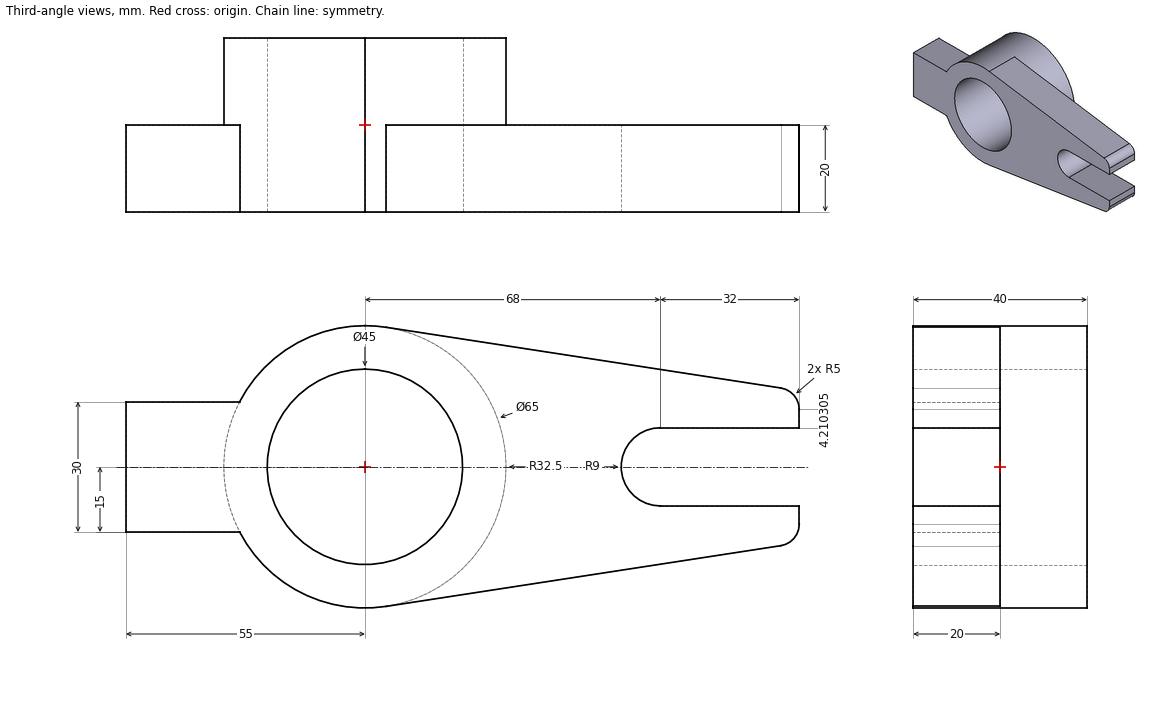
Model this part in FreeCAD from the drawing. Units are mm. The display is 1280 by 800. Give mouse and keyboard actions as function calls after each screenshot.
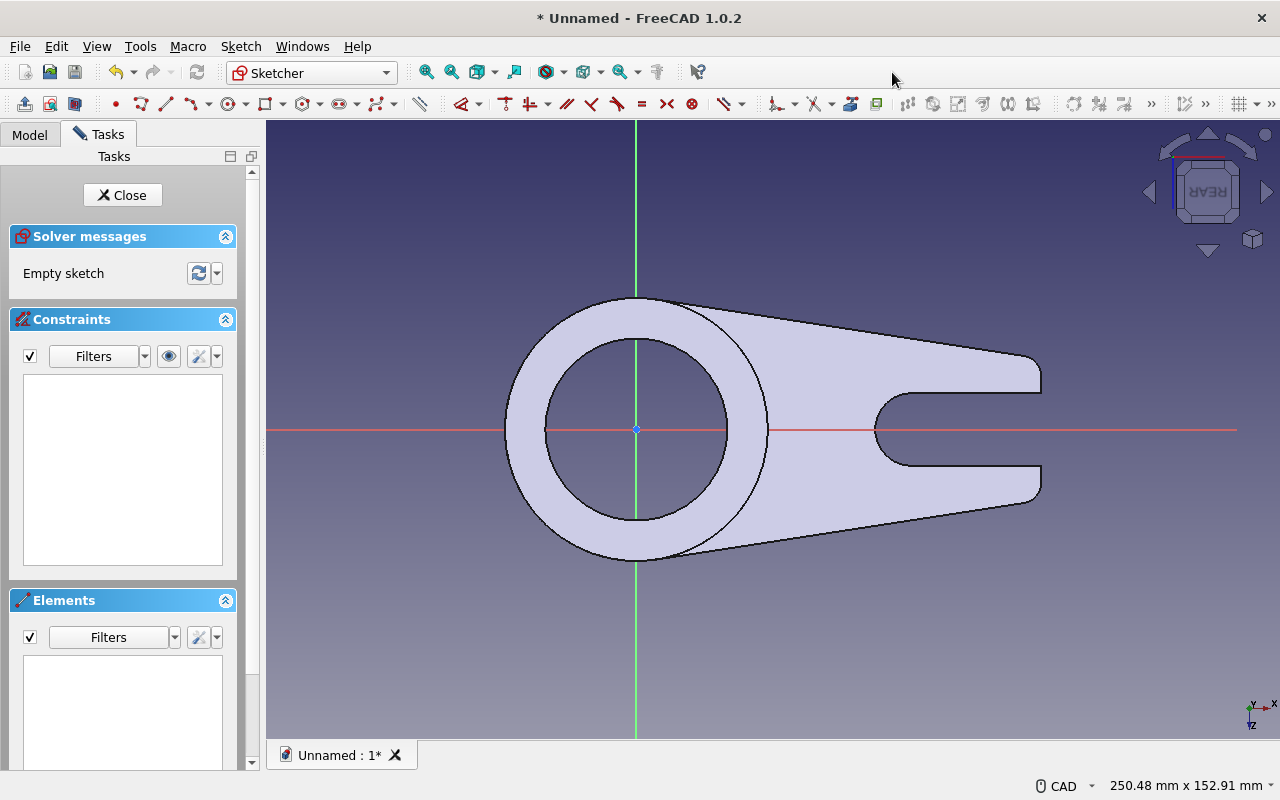
key(q)
key(s)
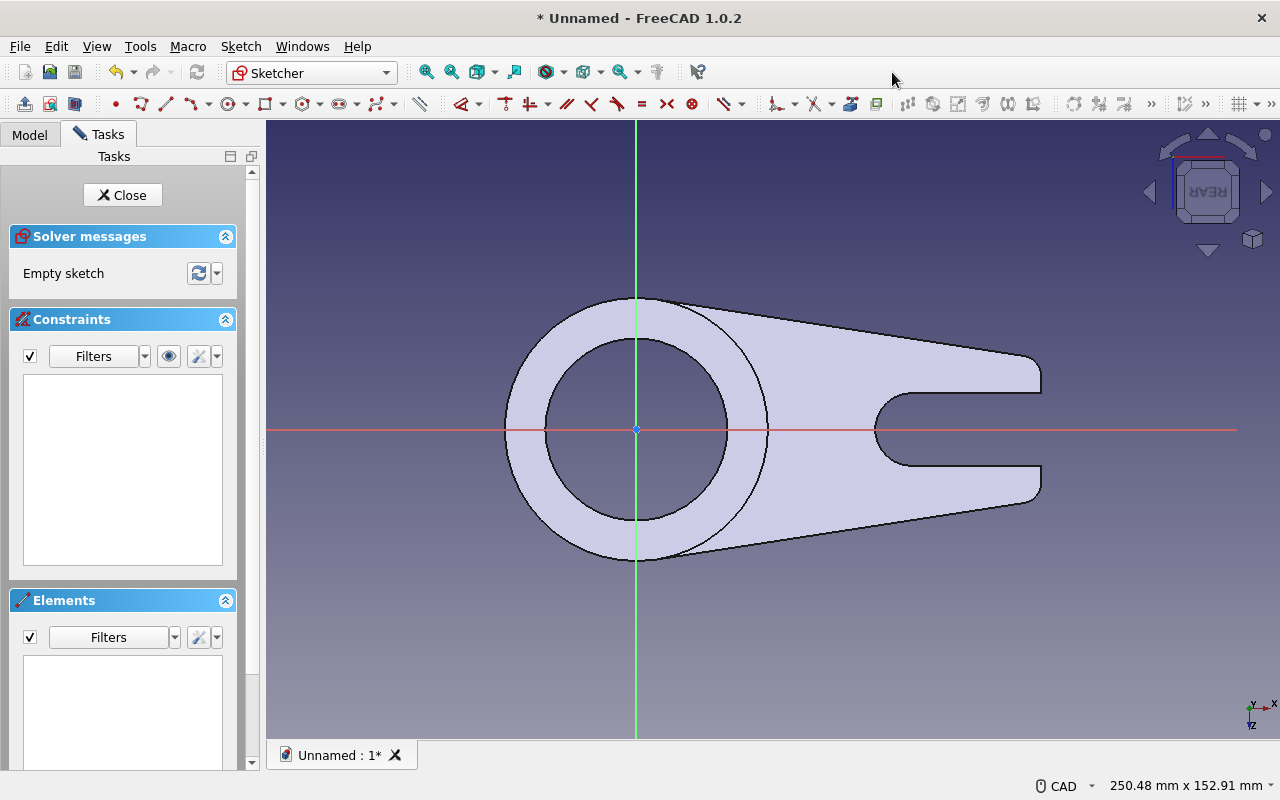
scroll(421, 429, up, 5)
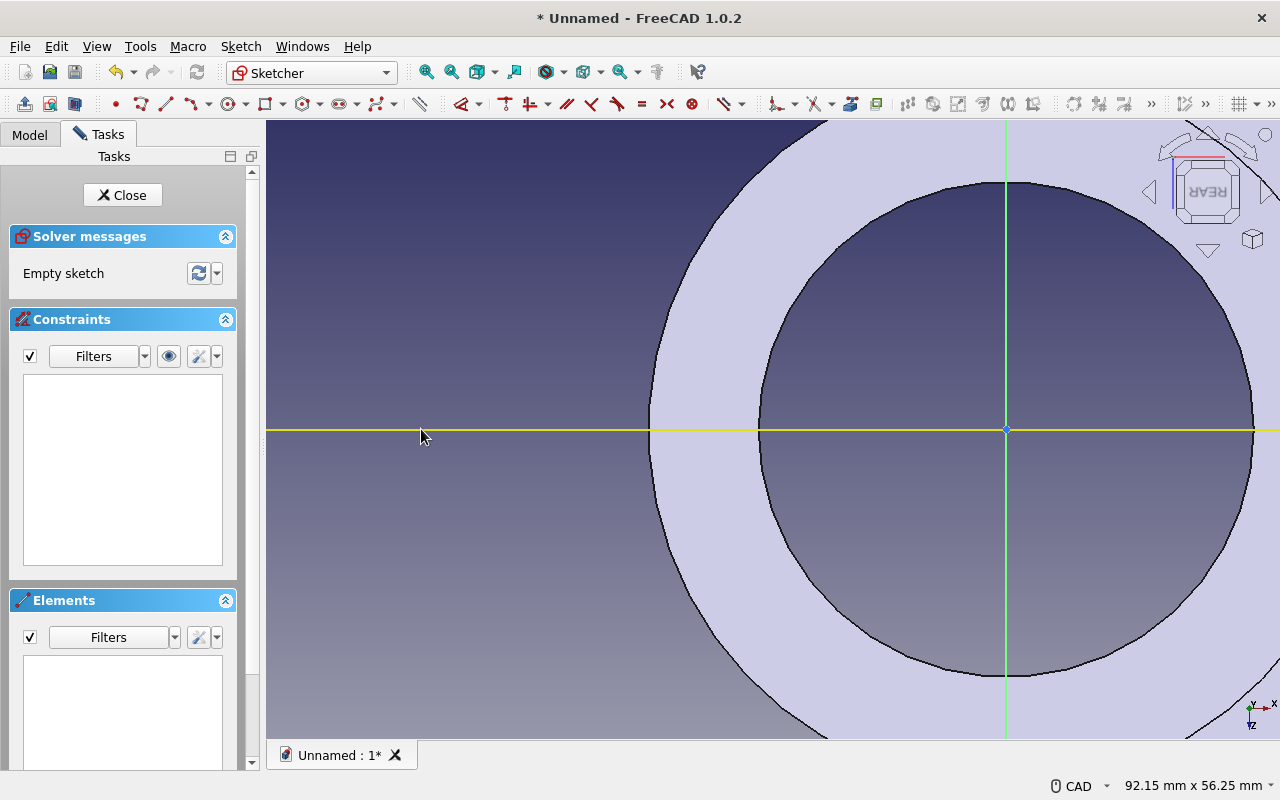
key(g)
key(m)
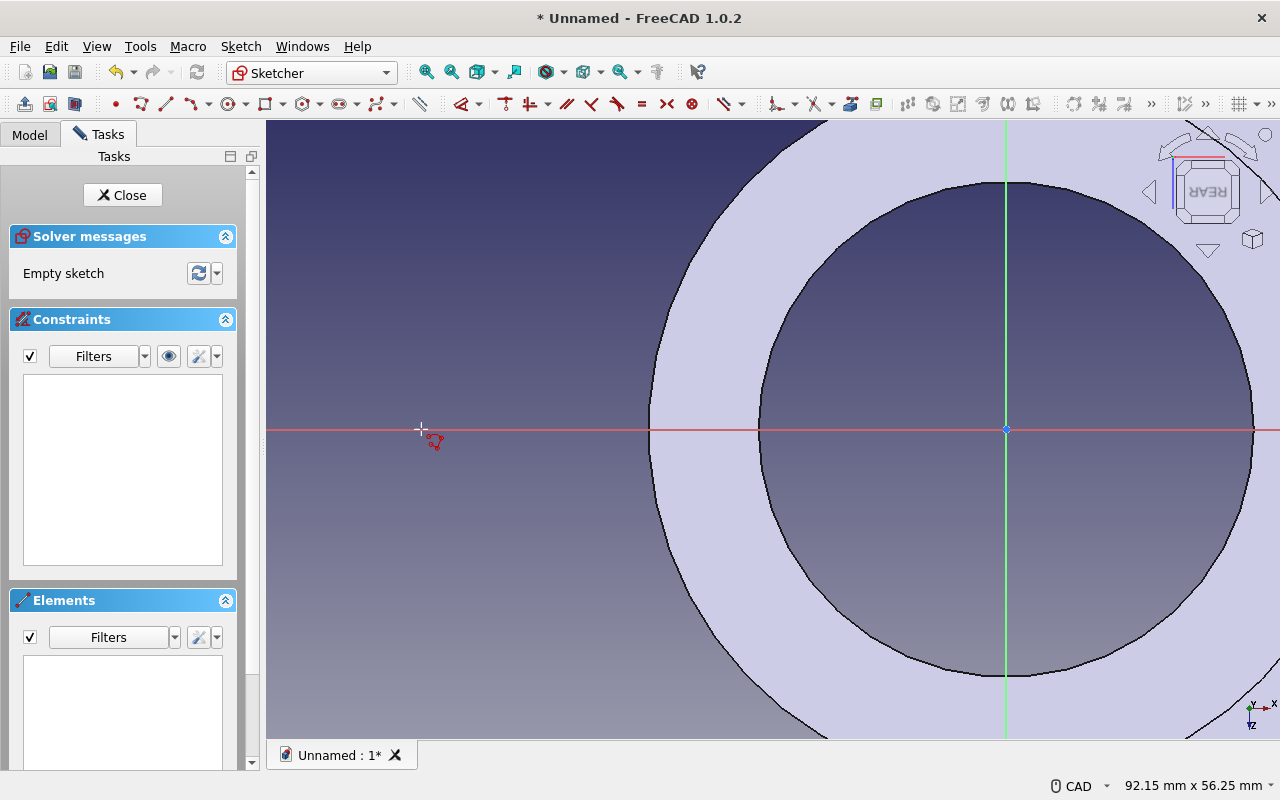
click(689, 264)
click(401, 264)
click(401, 595)
click(689, 595)
right_click(689, 595)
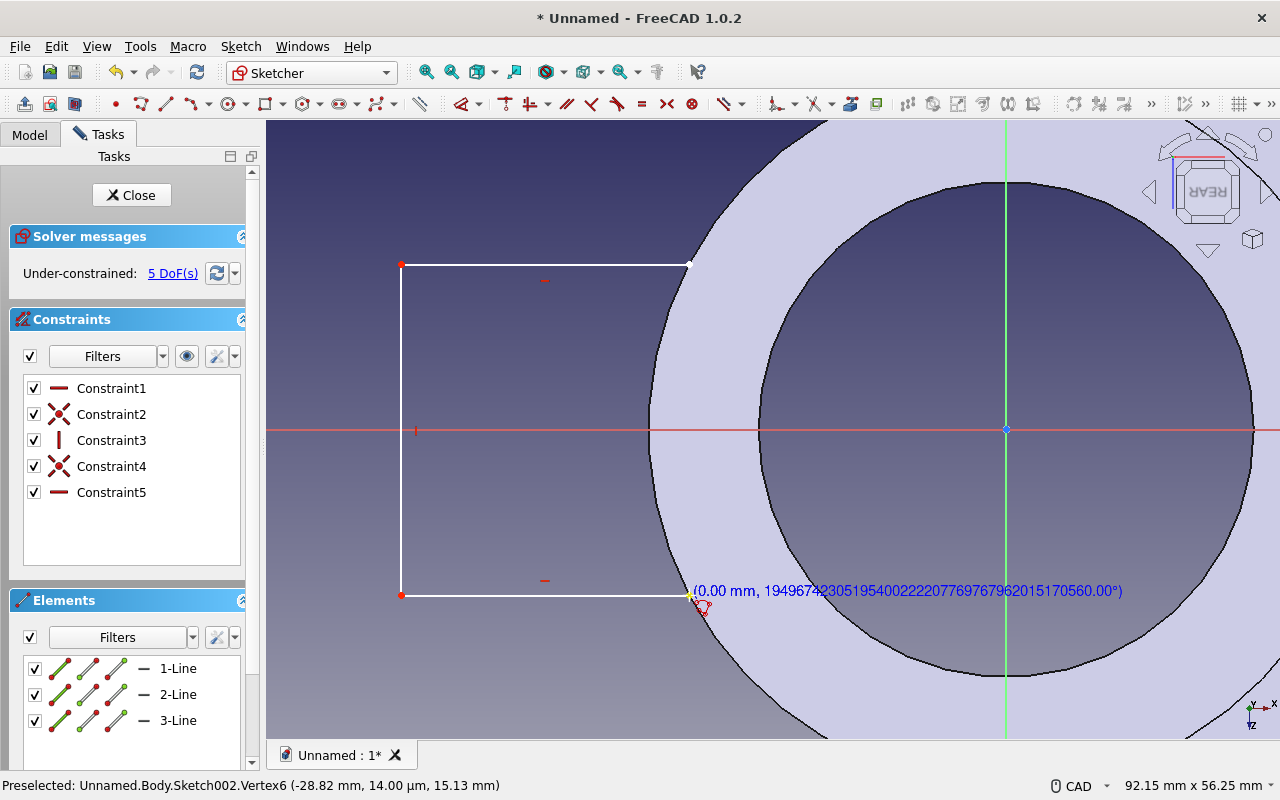
click(190, 104)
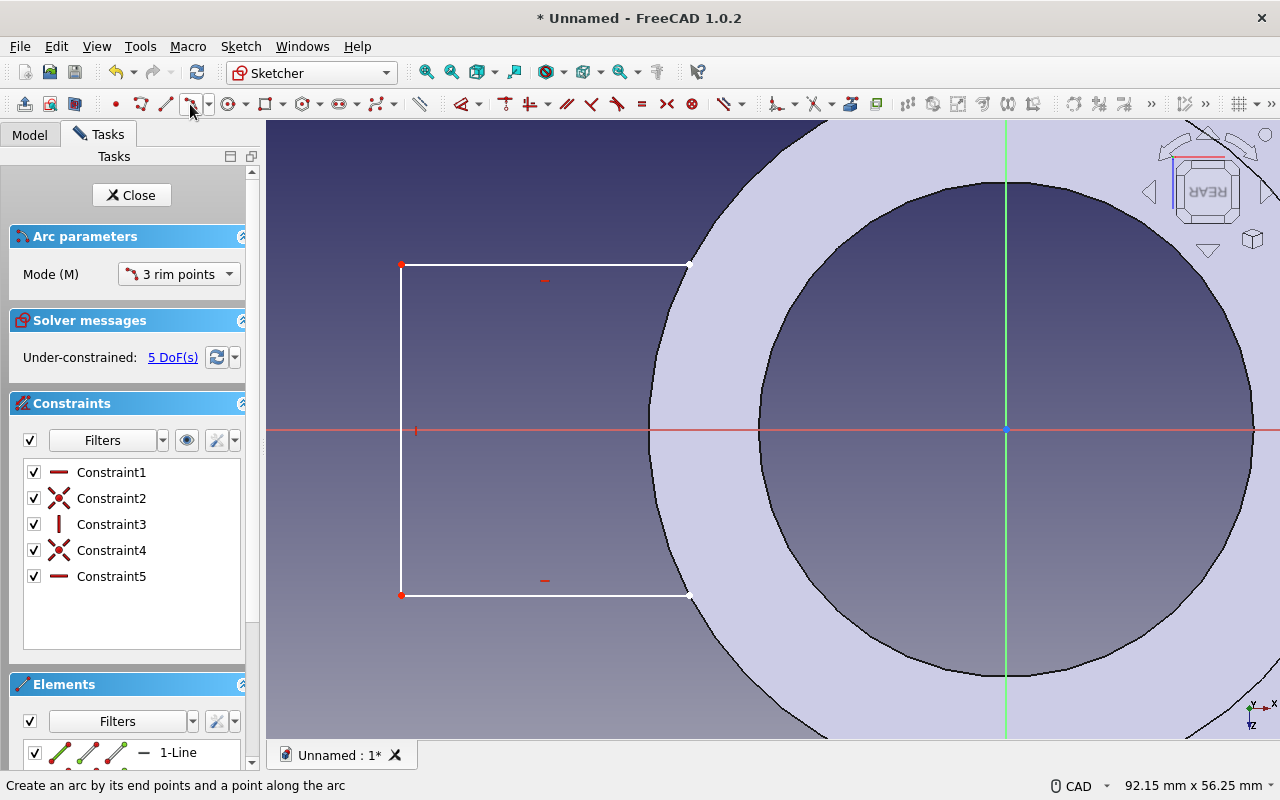
click(689, 596)
click(689, 265)
click(650, 395)
key(Escape)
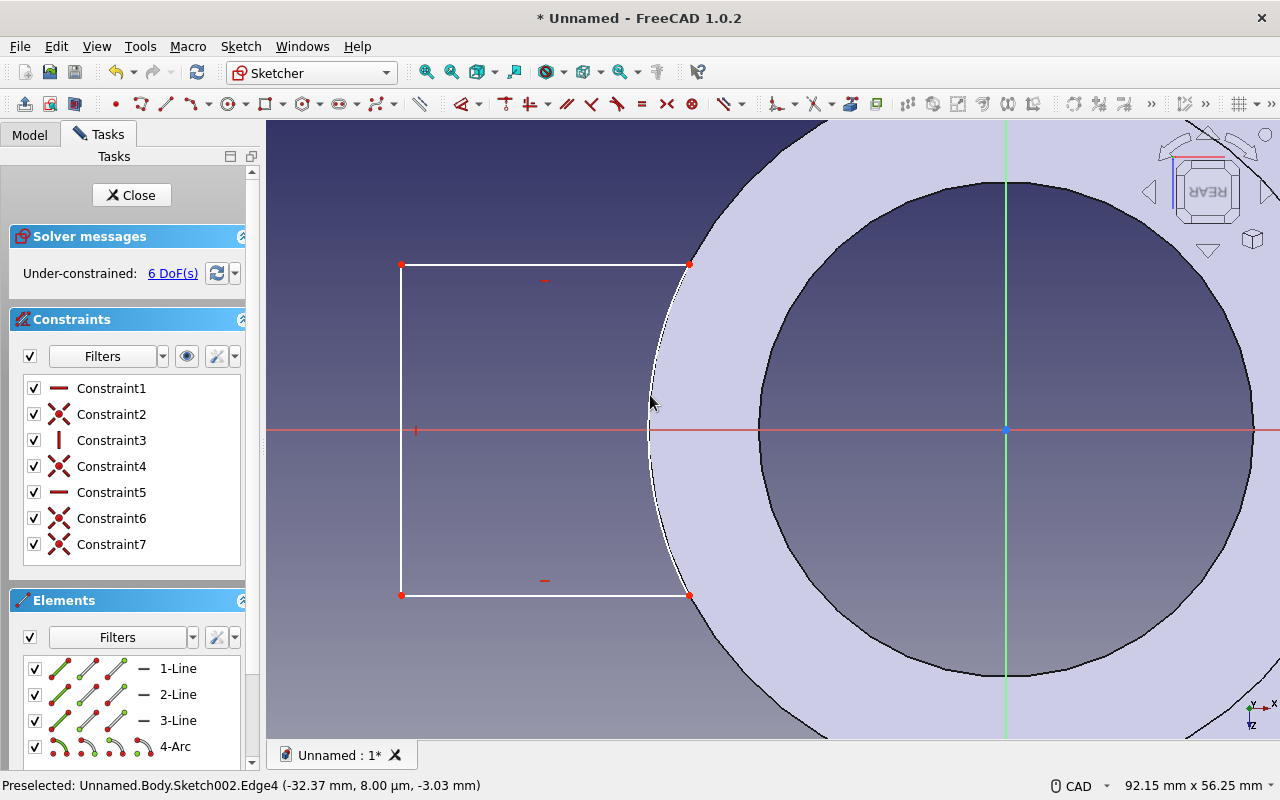
drag(995, 419, 1016, 441)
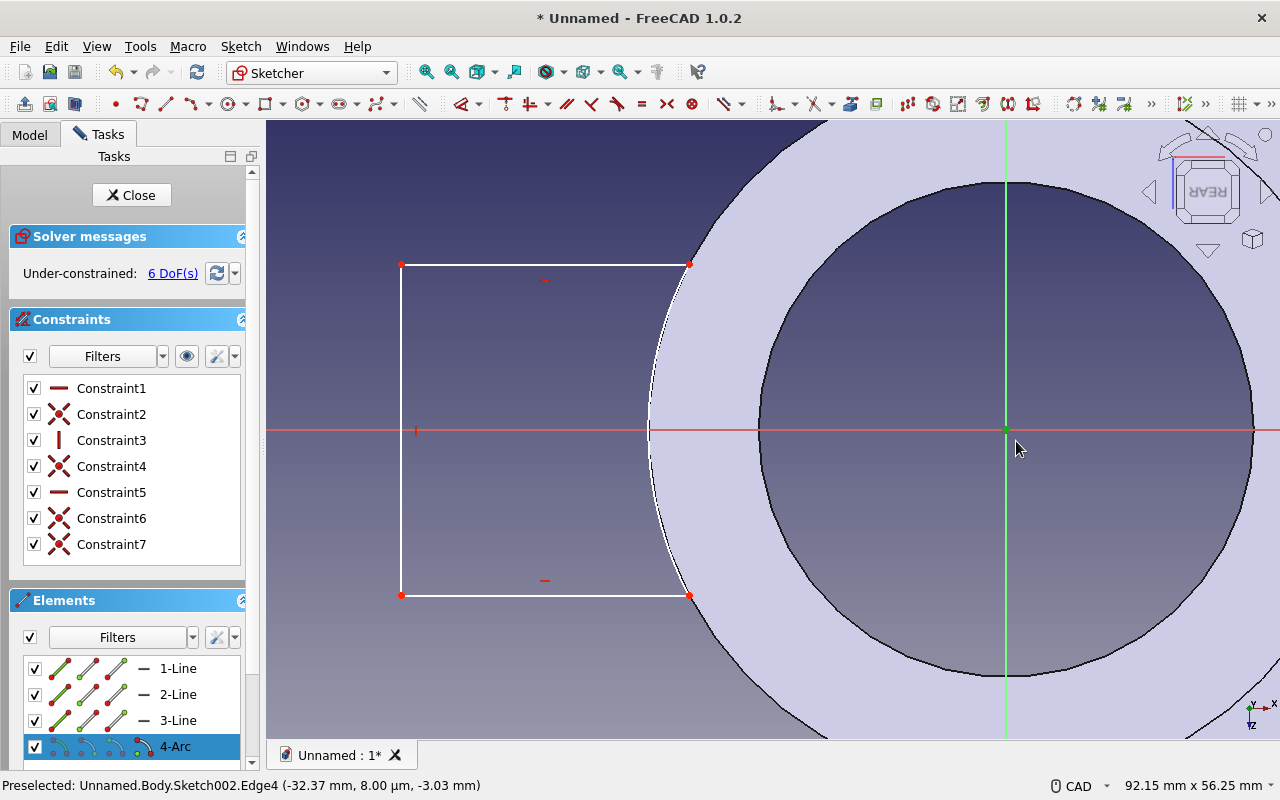
key(c)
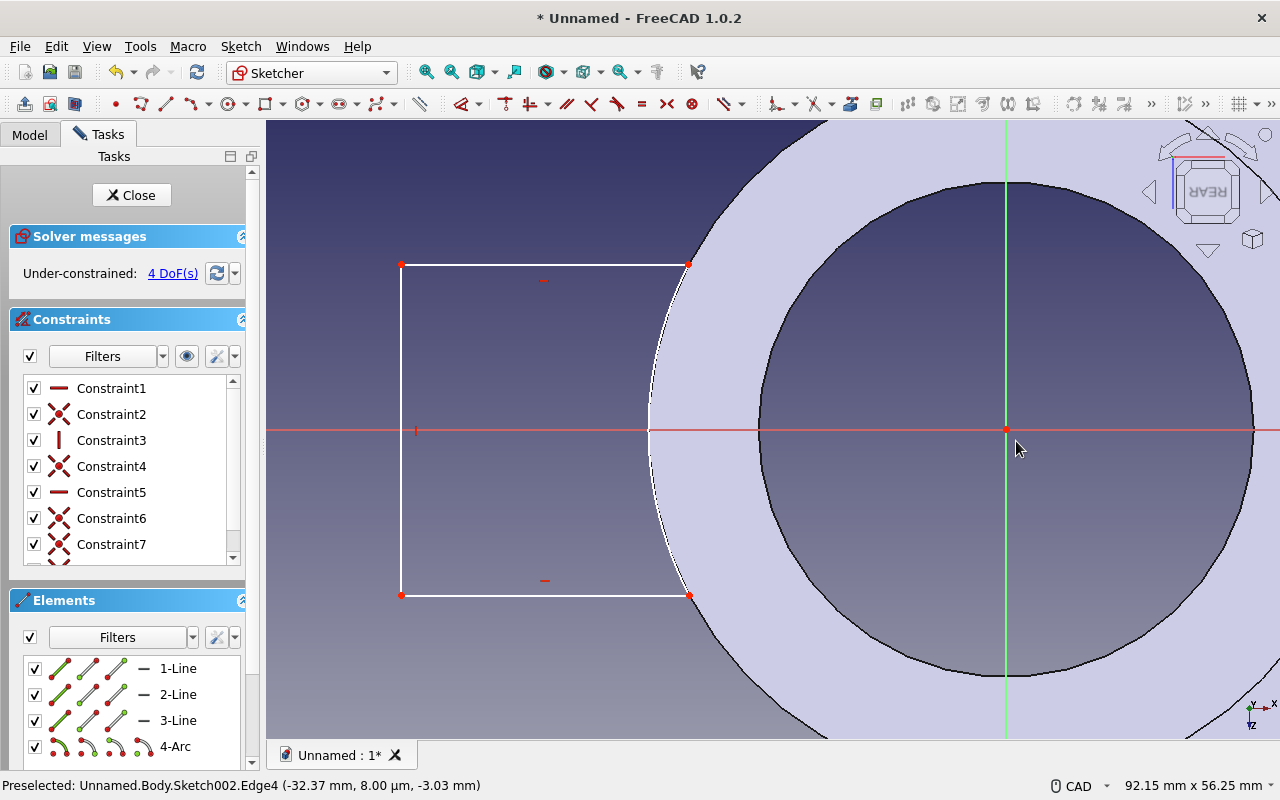
key(d)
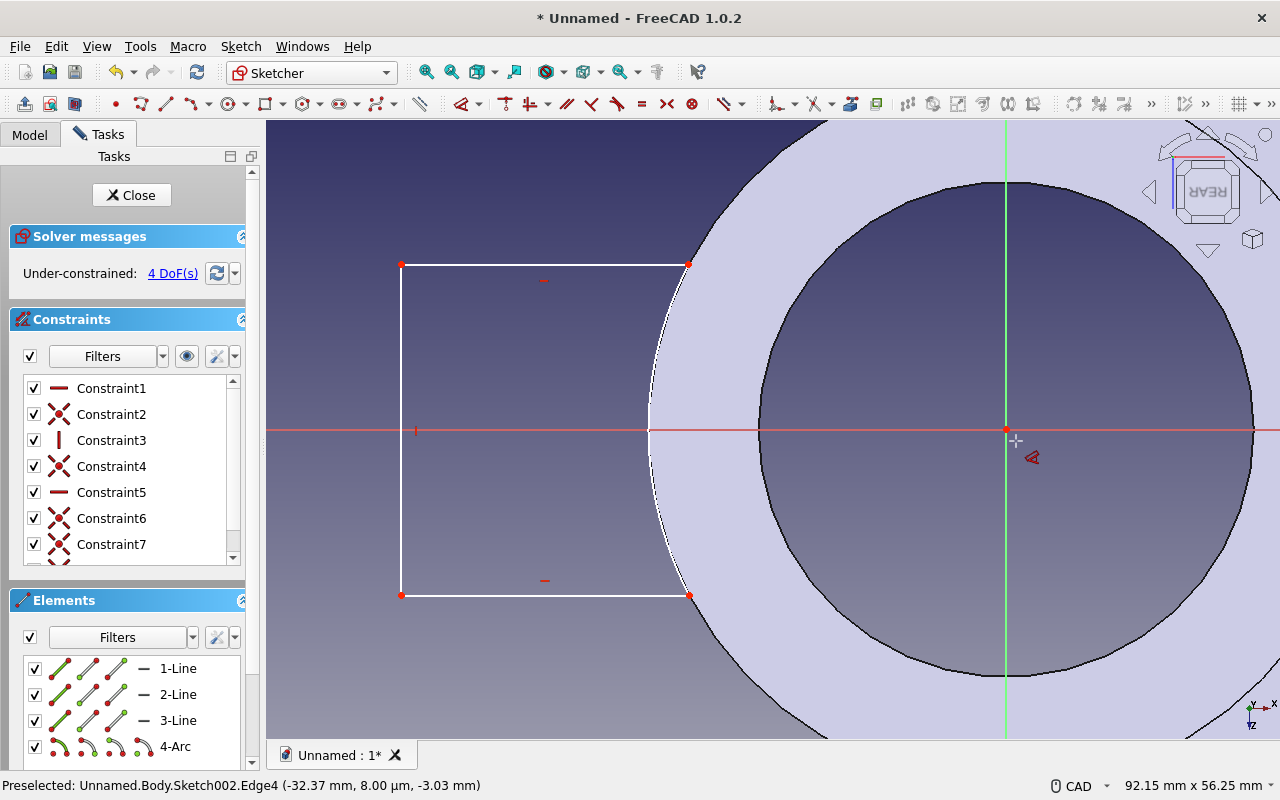
click(655, 362)
click(624, 356)